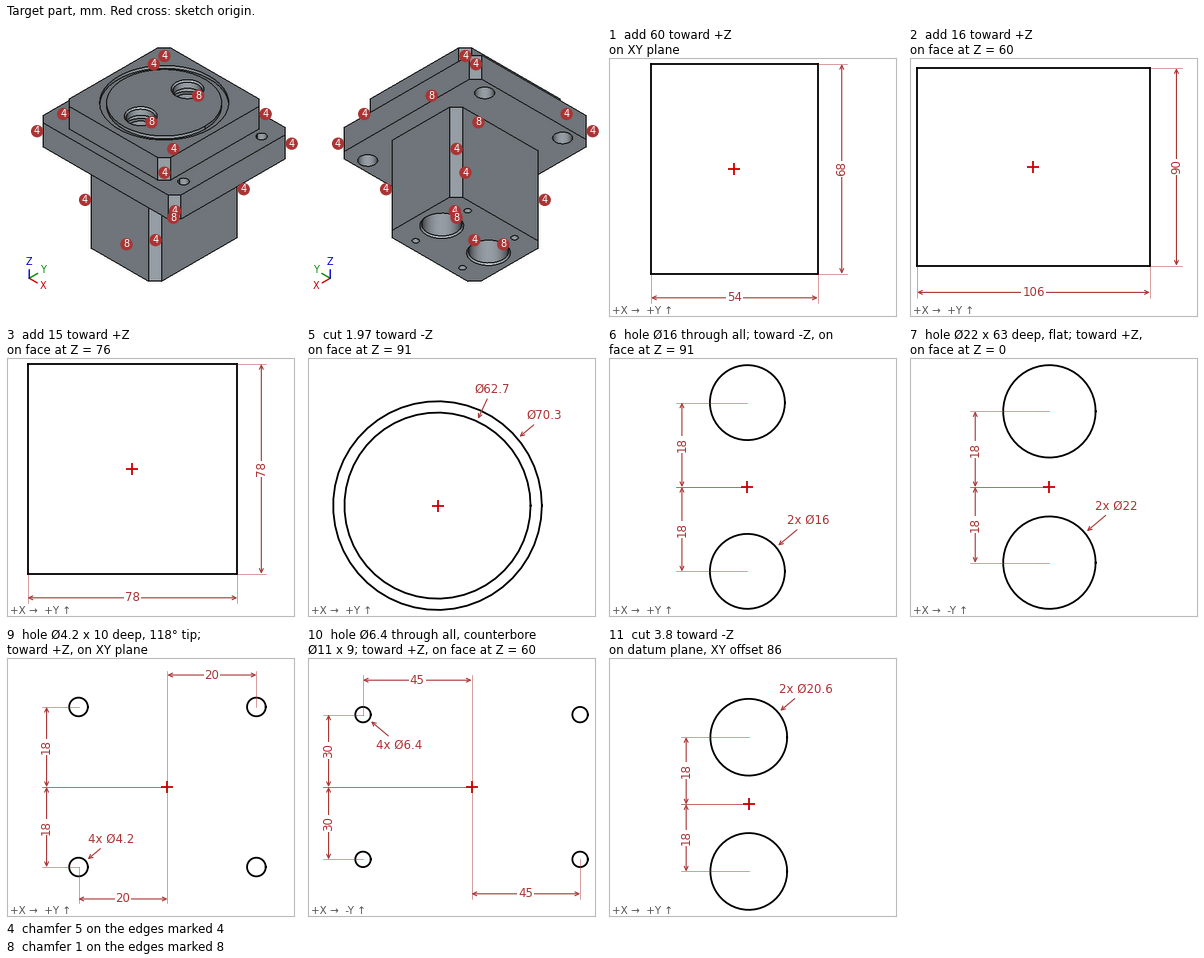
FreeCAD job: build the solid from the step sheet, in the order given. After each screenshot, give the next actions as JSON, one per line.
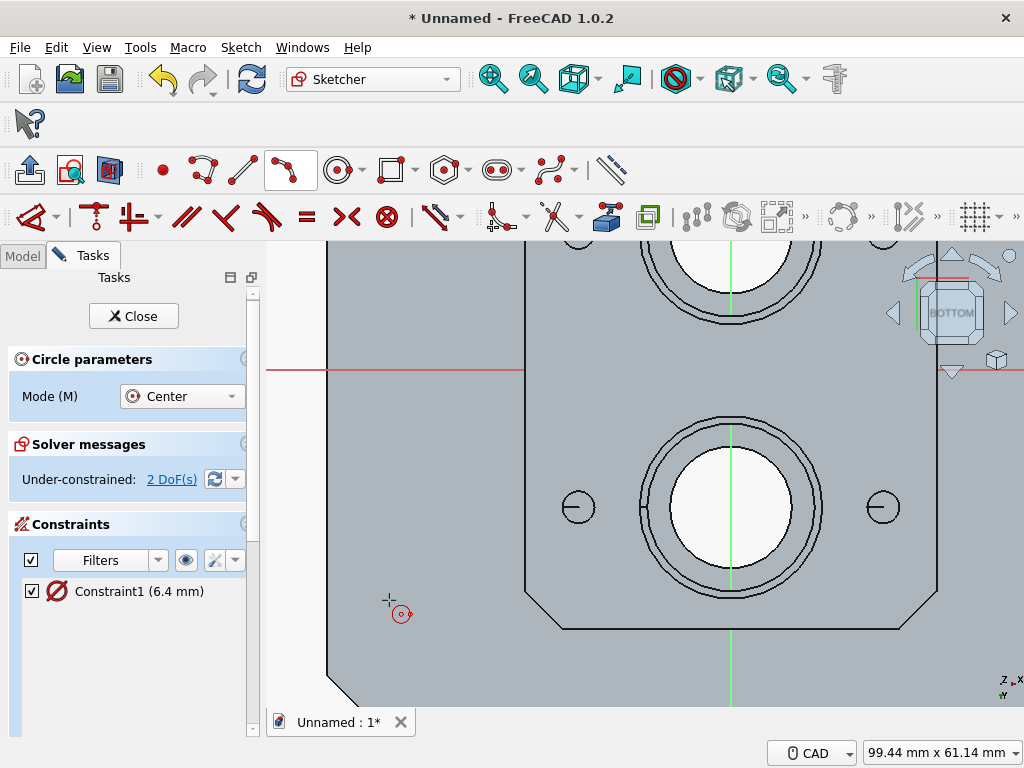
{"action": "left_click", "coordinate": [388, 599]}
{"action": "mouse_move", "coordinate": [405, 582]}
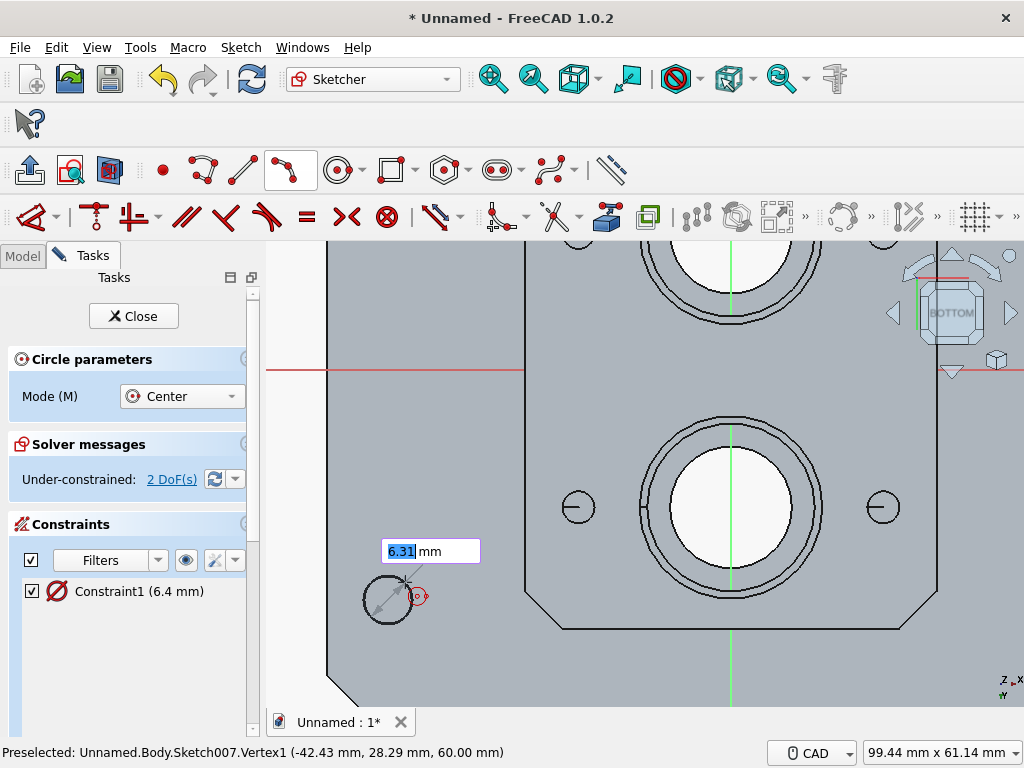
{"action": "type", "text": "6.4"}
{"action": "key", "text": "Return"}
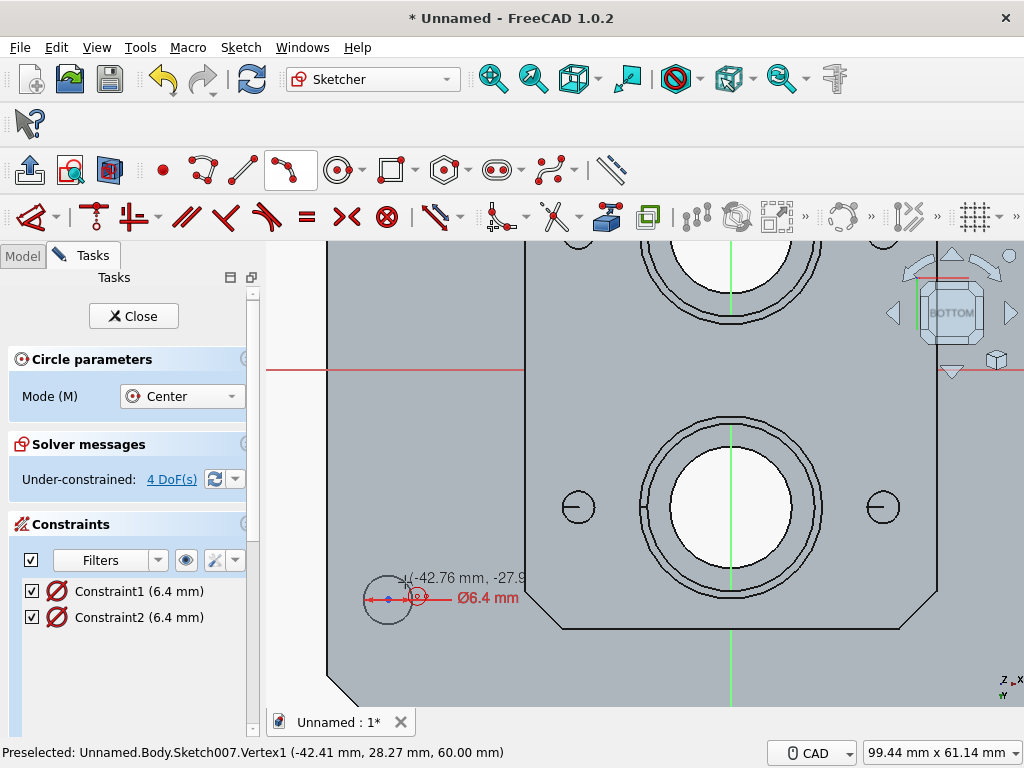
{"action": "scroll", "coordinate": [389, 600], "scroll_direction": "down", "scroll_amount": 3}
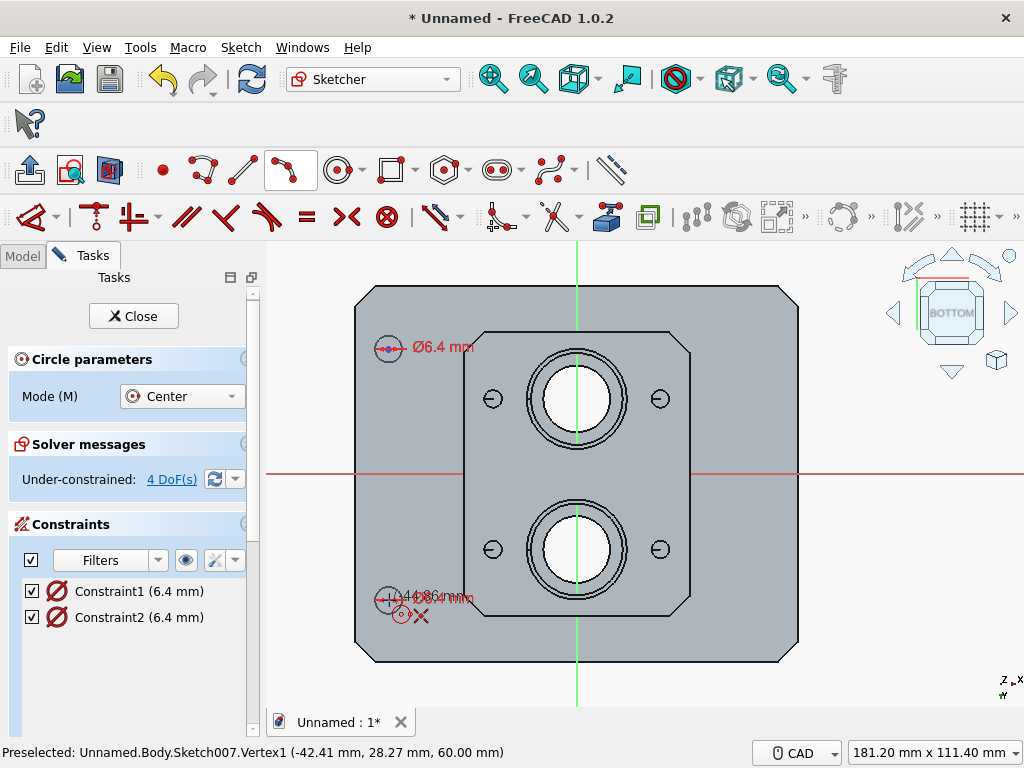
{"action": "scroll", "coordinate": [765, 600], "scroll_direction": "up", "scroll_amount": 3}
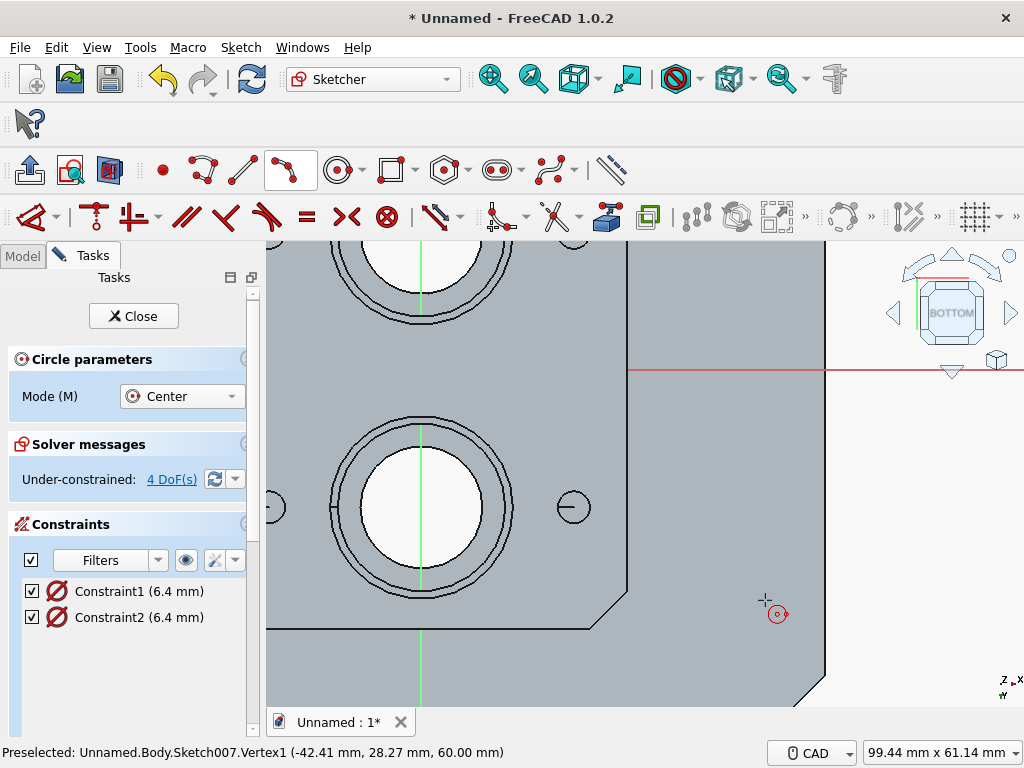
{"action": "left_click", "coordinate": [764, 599]}
{"action": "mouse_move", "coordinate": [782, 582]}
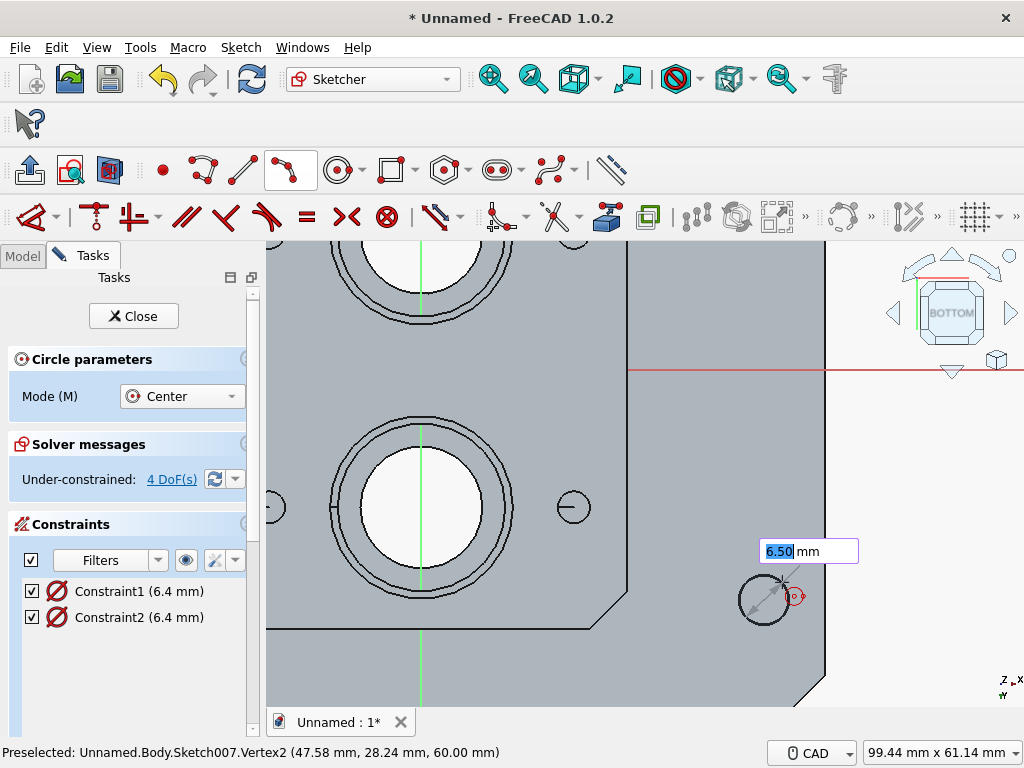
{"action": "type", "text": "6.4"}
{"action": "key", "text": "Return"}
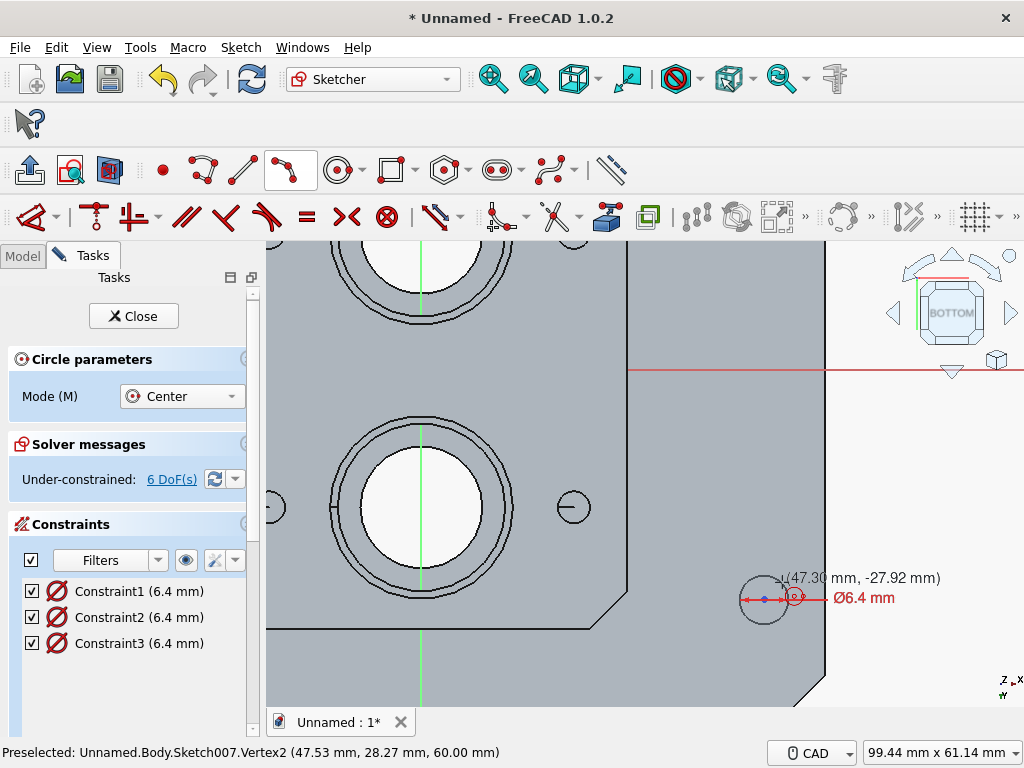
{"action": "scroll", "coordinate": [765, 600], "scroll_direction": "down", "scroll_amount": 3}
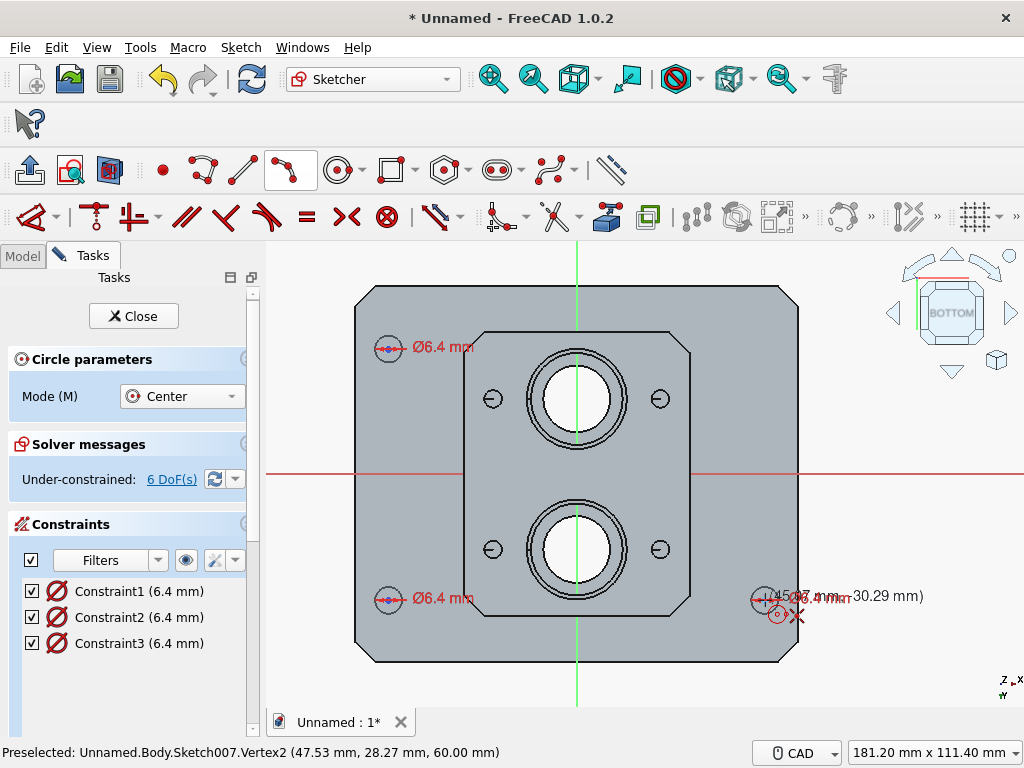
{"action": "scroll", "coordinate": [765, 349], "scroll_direction": "up", "scroll_amount": 3}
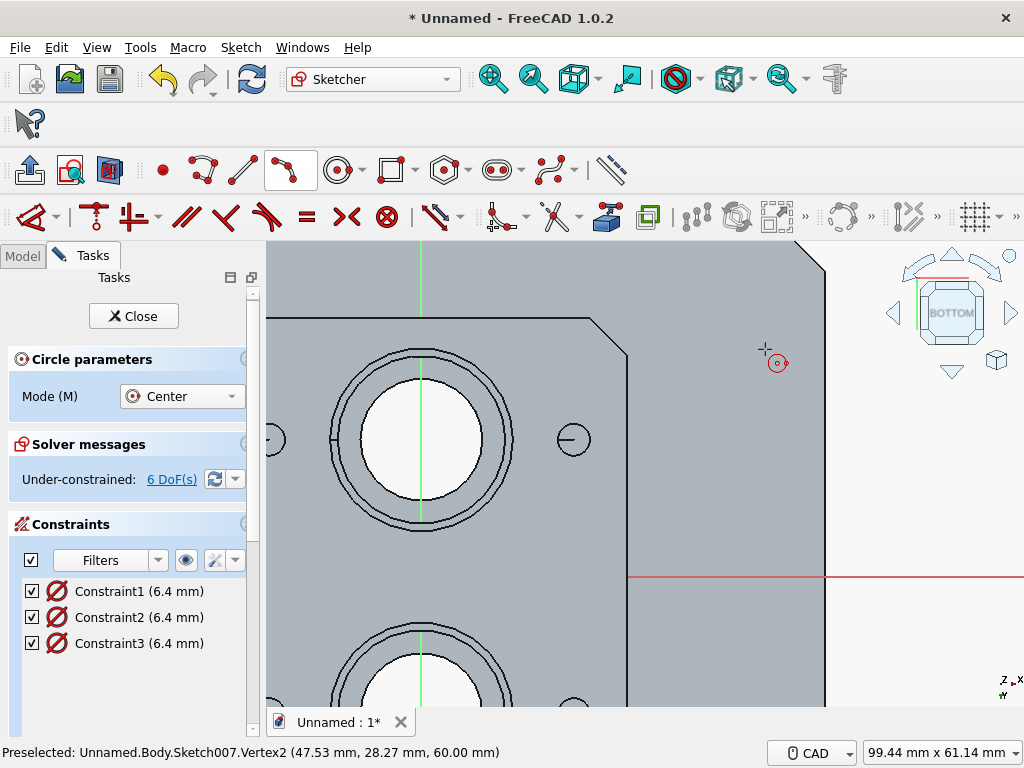
{"action": "left_click", "coordinate": [764, 348]}
{"action": "mouse_move", "coordinate": [782, 331]}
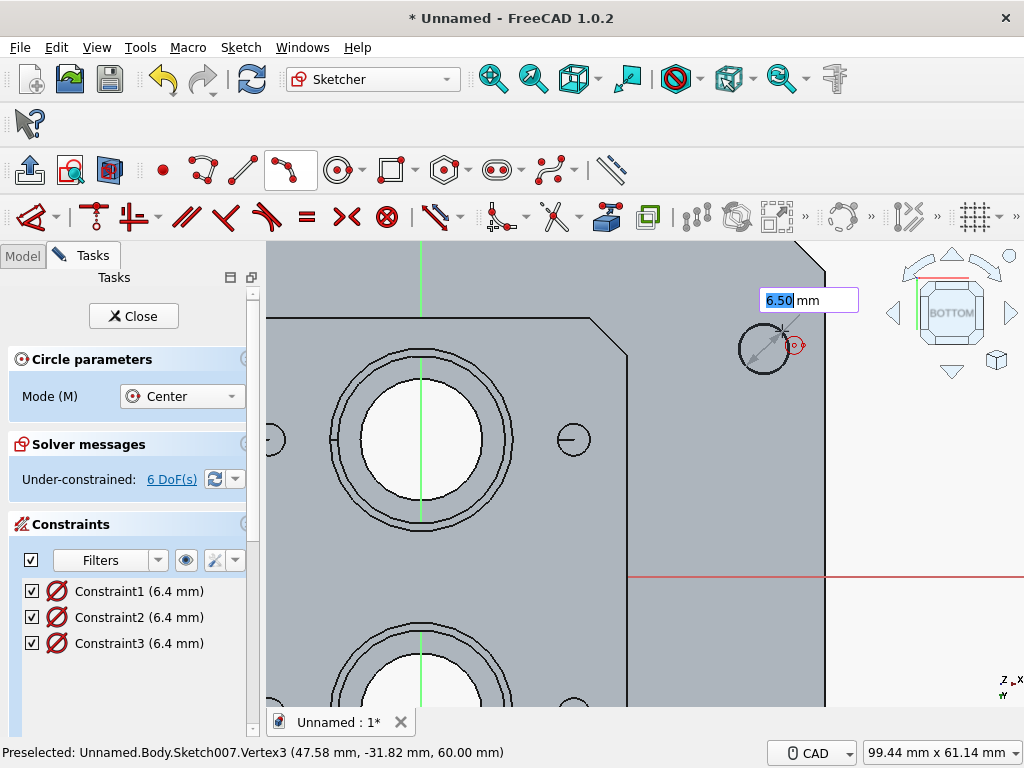
{"action": "type", "text": "6.4"}
{"action": "key", "text": "Return"}
{"action": "key", "text": "Escape"}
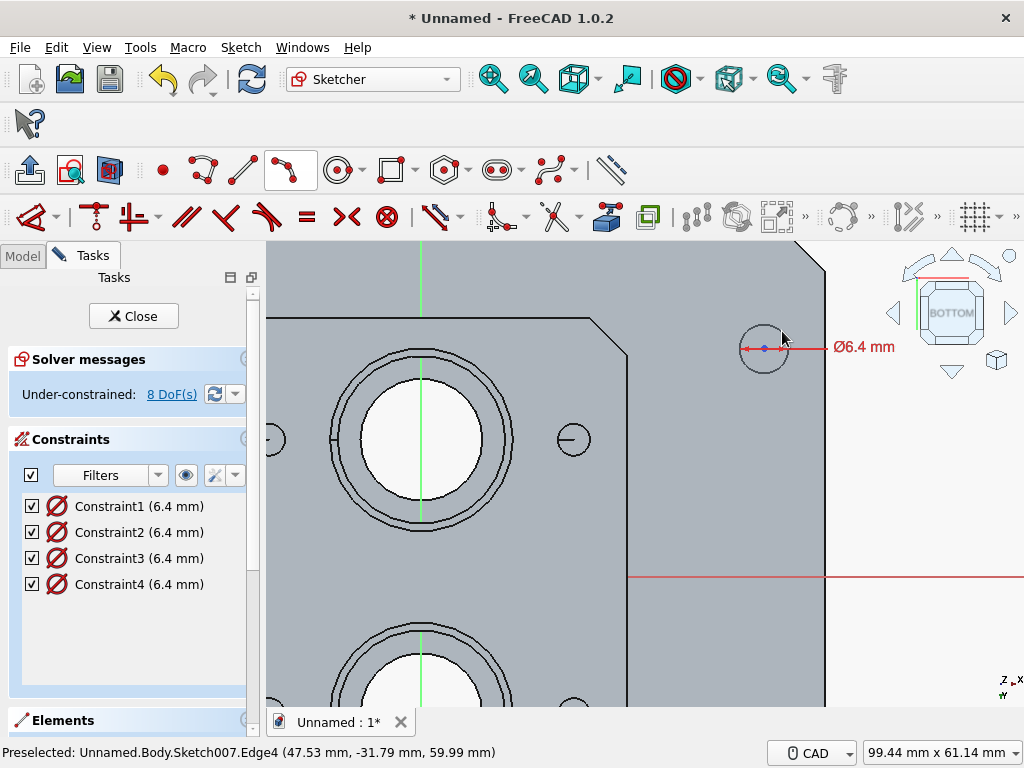
{"action": "scroll", "coordinate": [765, 349], "scroll_direction": "down", "scroll_amount": 3}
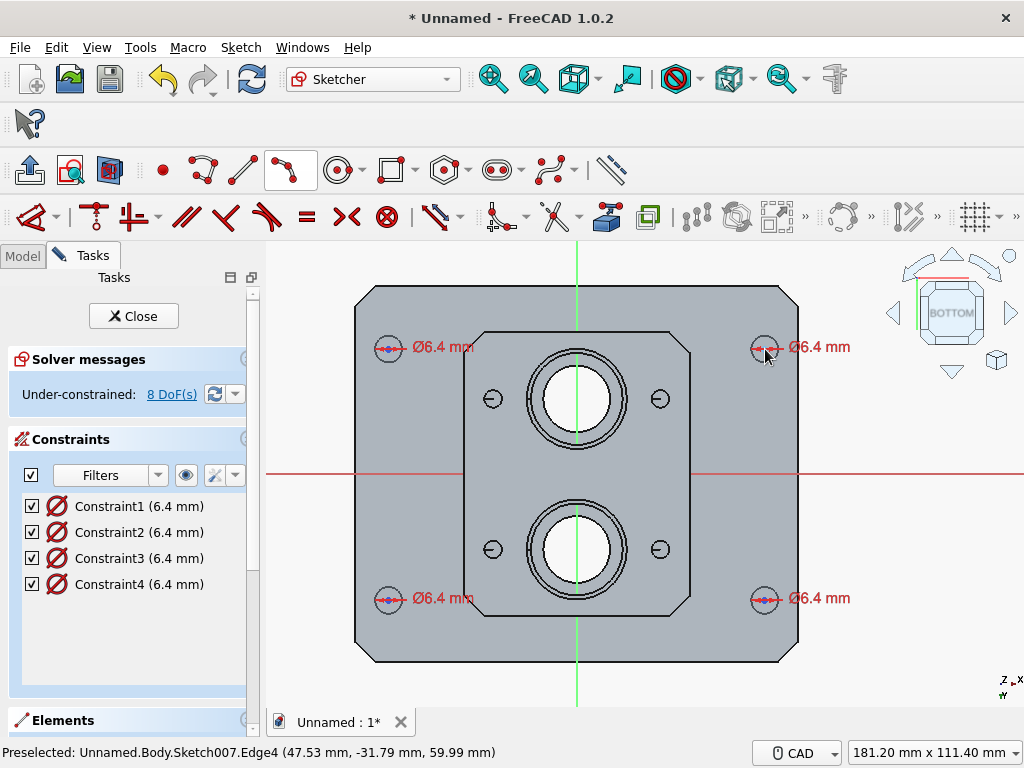
{"action": "left_click", "coordinate": [389, 349]}